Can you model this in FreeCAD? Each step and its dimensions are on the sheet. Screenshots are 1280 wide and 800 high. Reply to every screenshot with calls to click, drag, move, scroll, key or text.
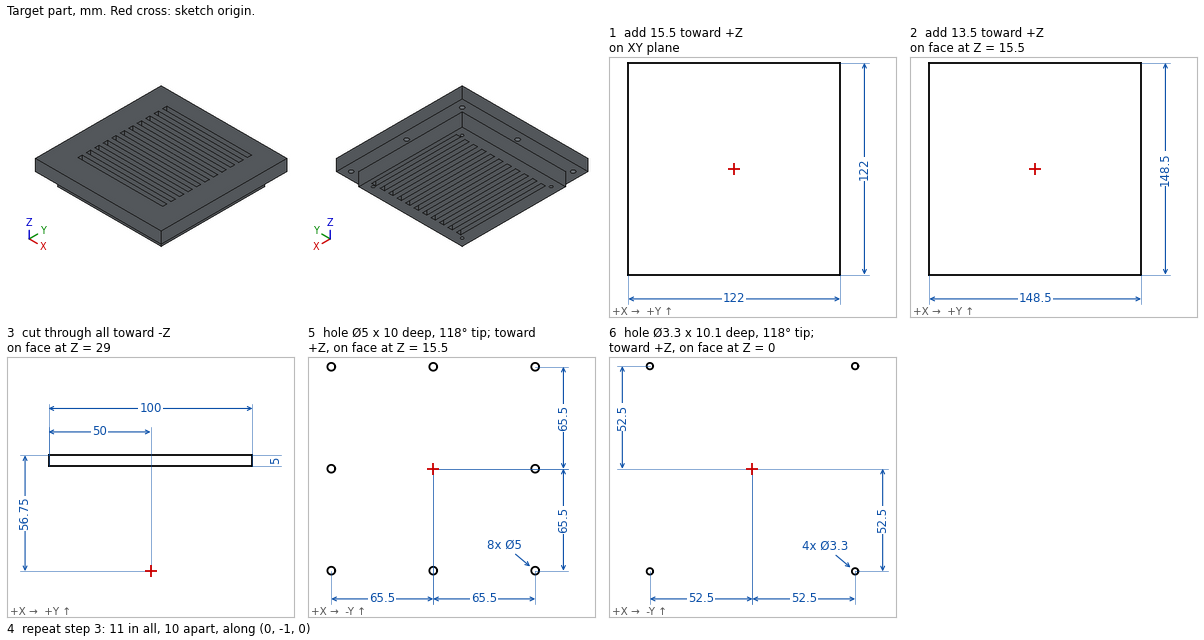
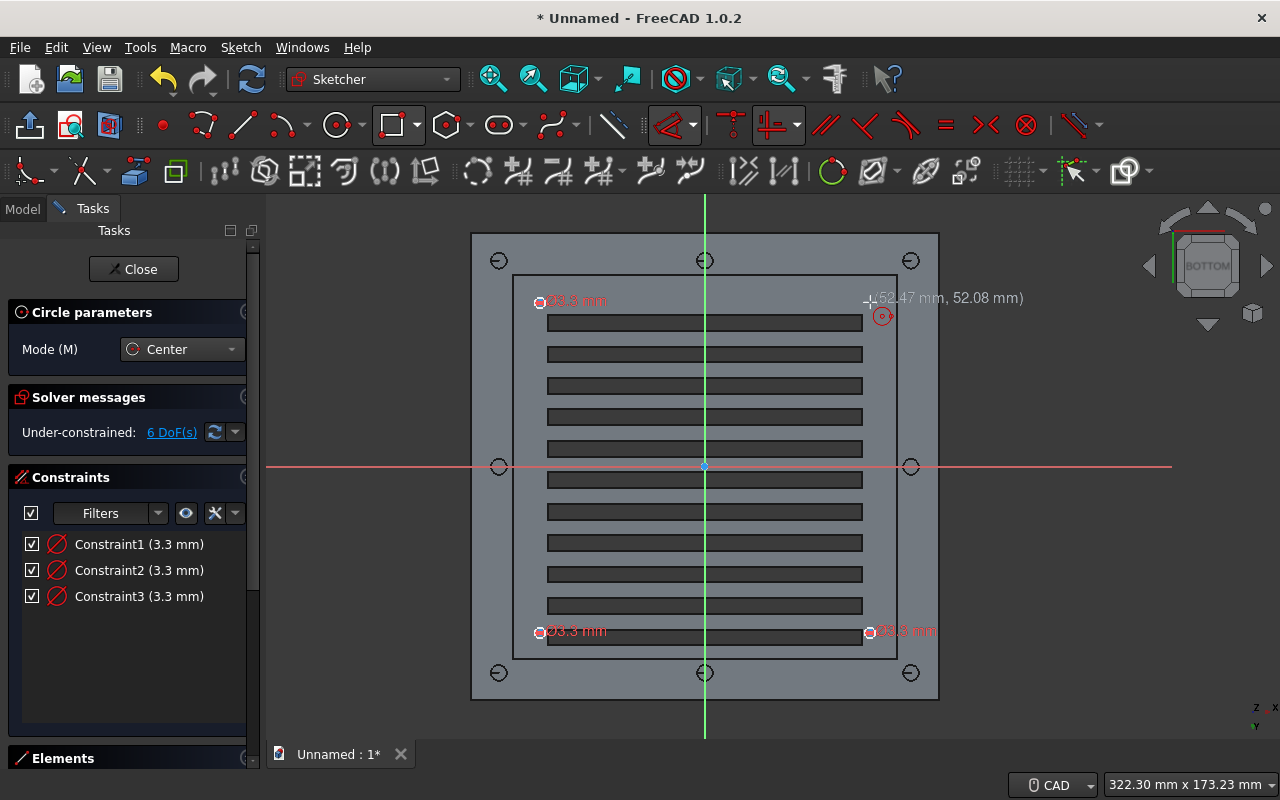
click(870, 302)
move(874, 298)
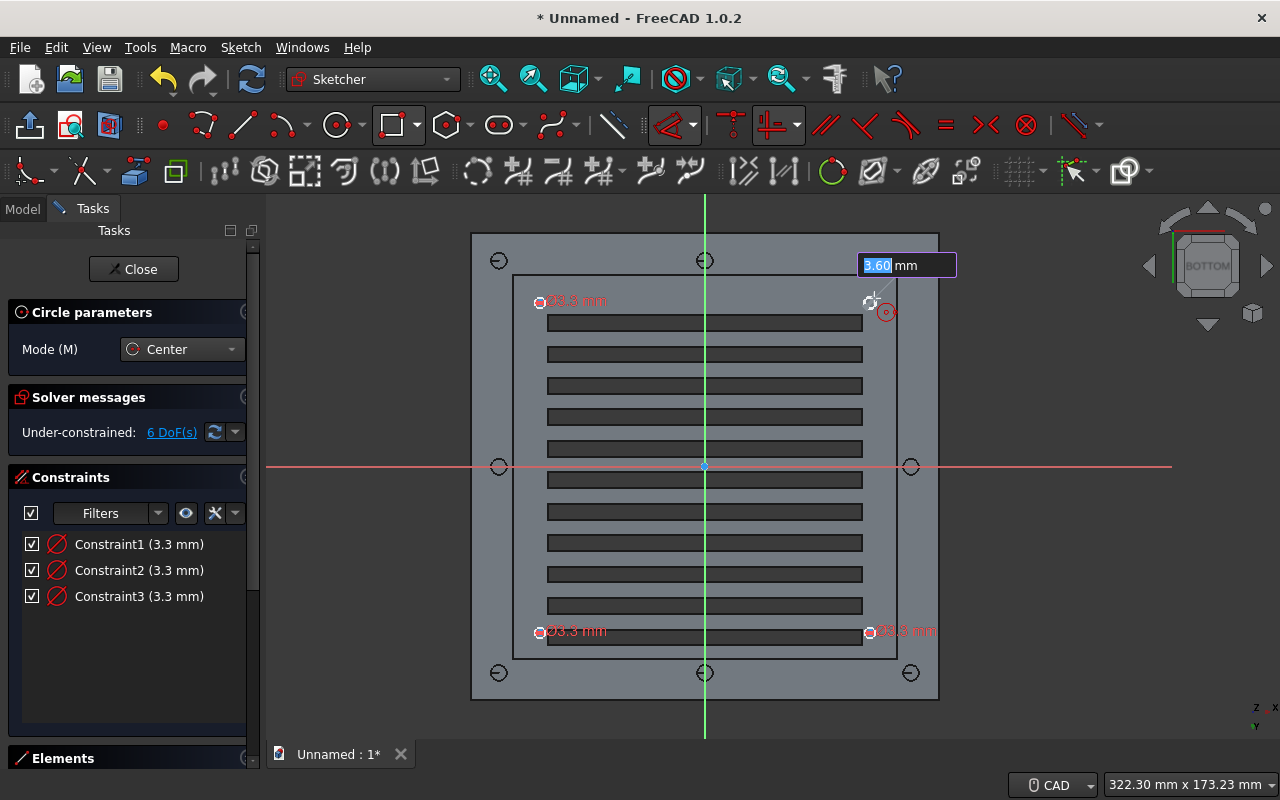
text(3.3)
key(Return)
key(Escape)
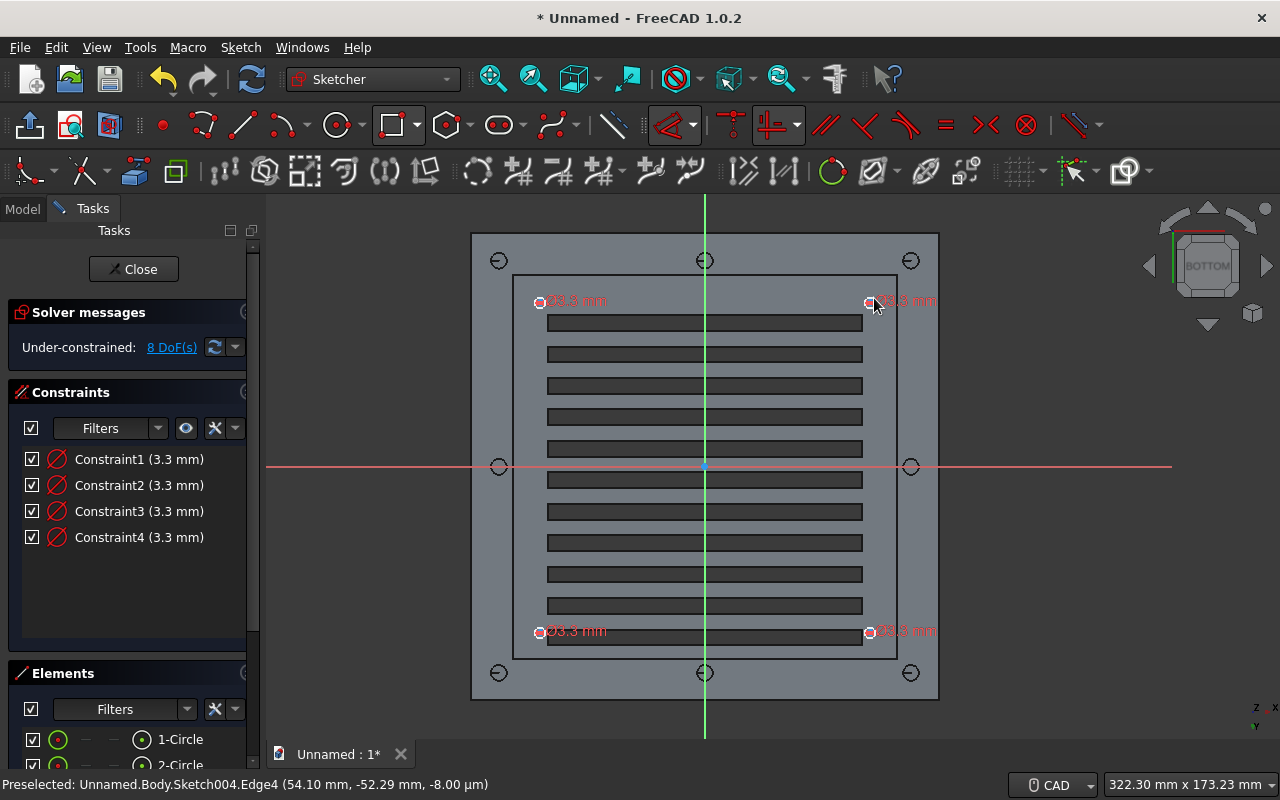
click(870, 633)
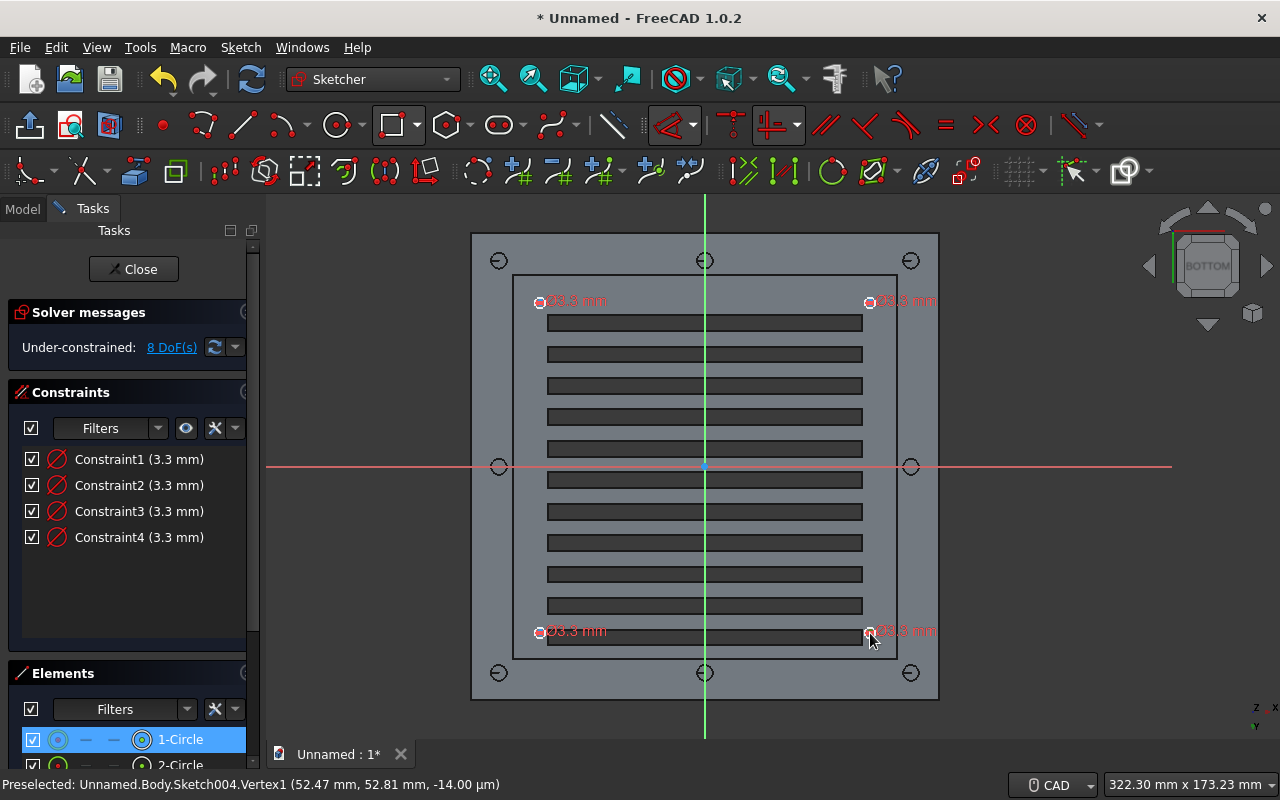
click(540, 633)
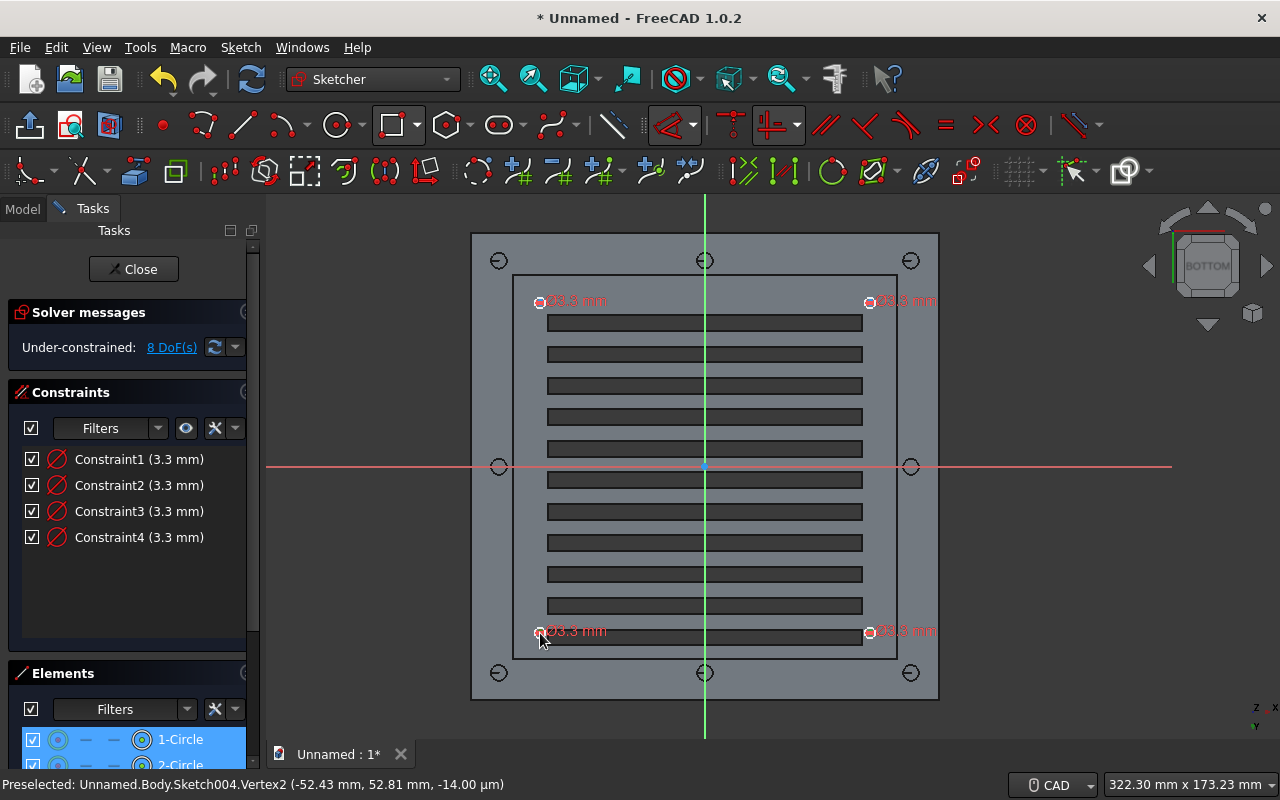
click(800, 126)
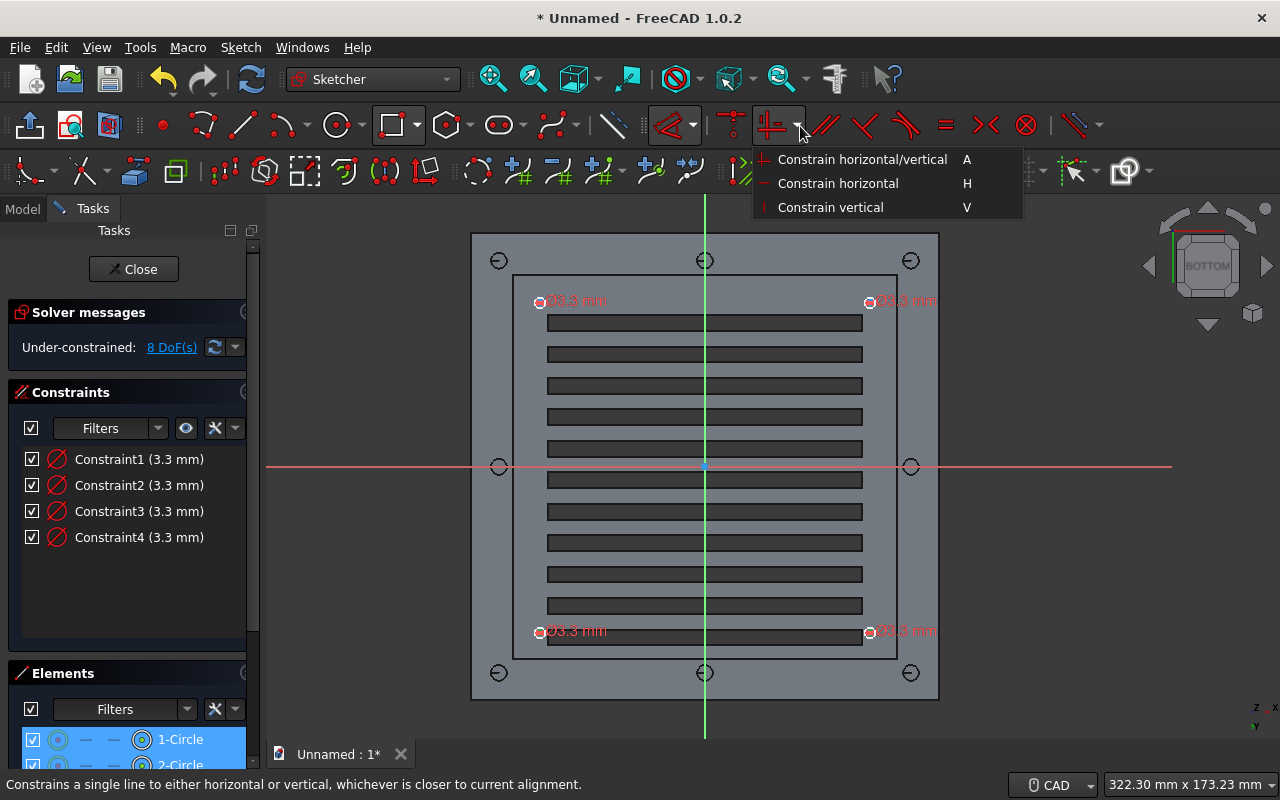
click(888, 183)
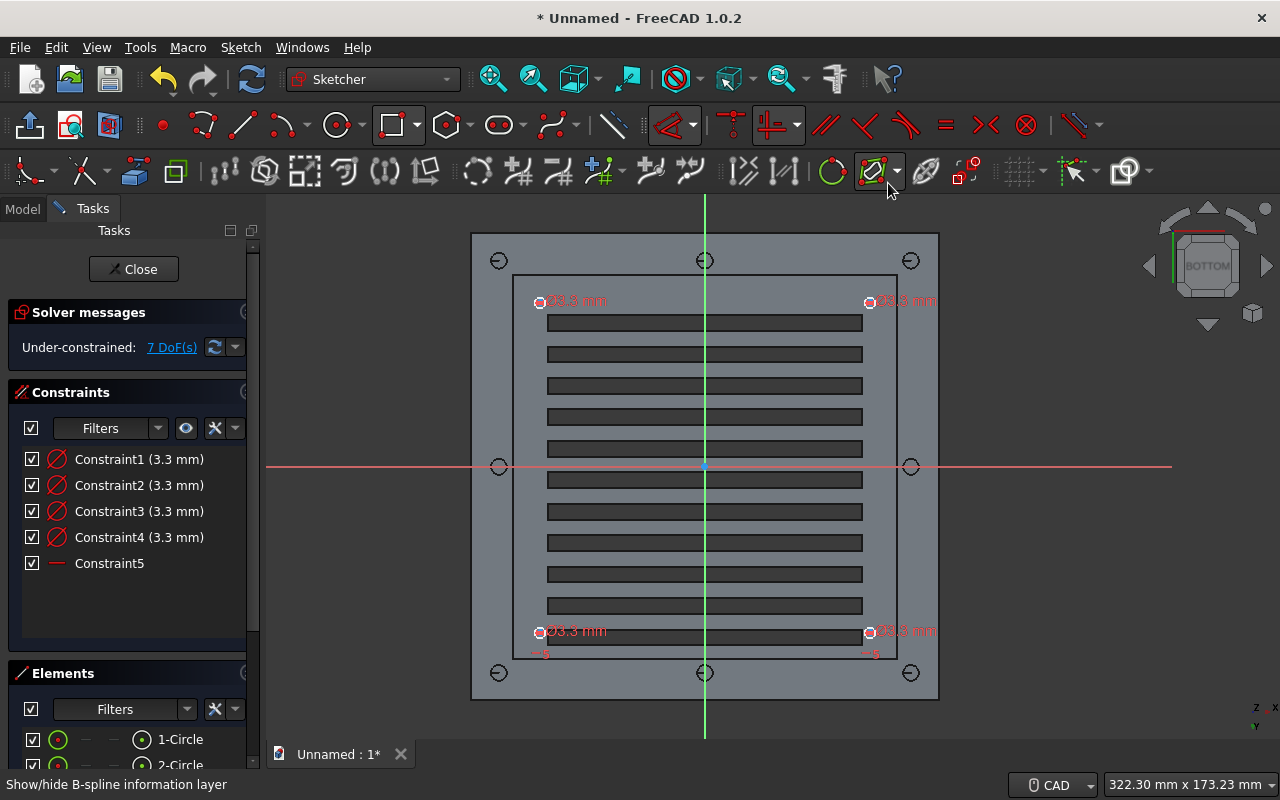
click(540, 633)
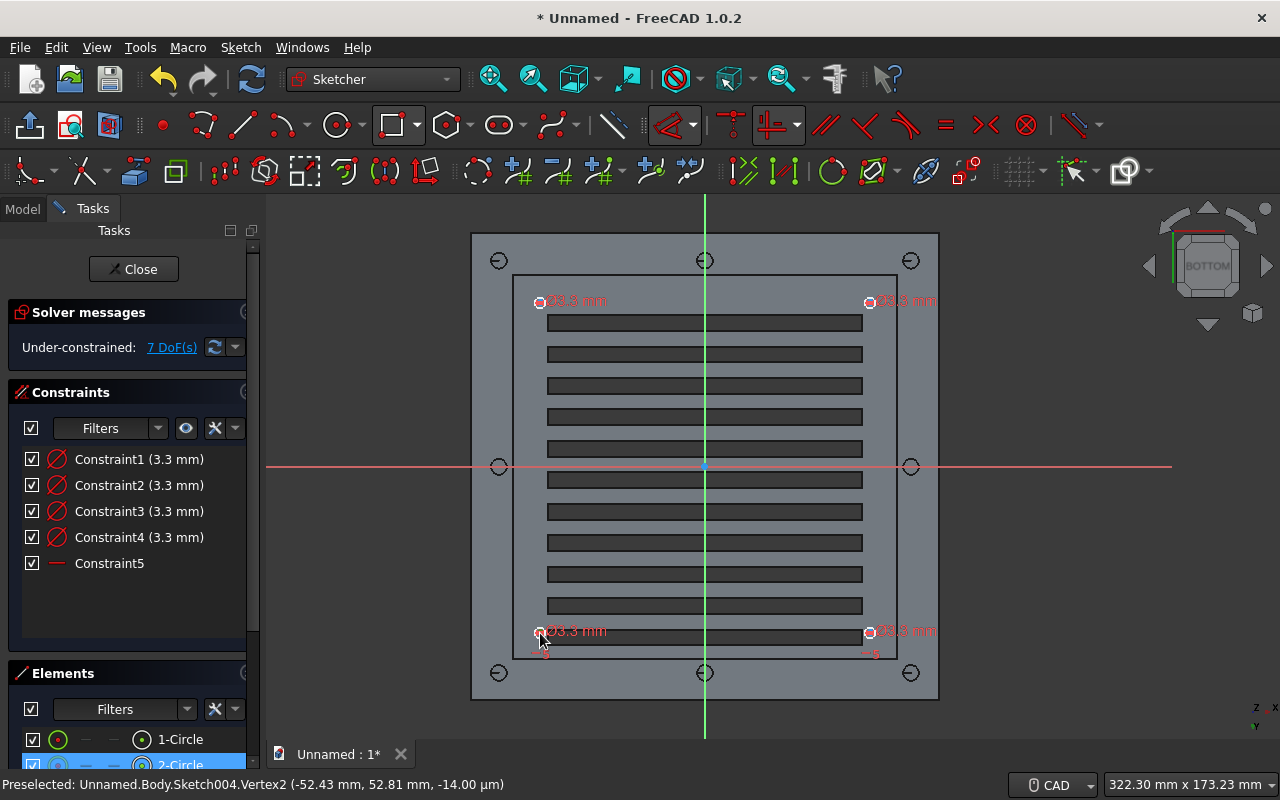
click(540, 303)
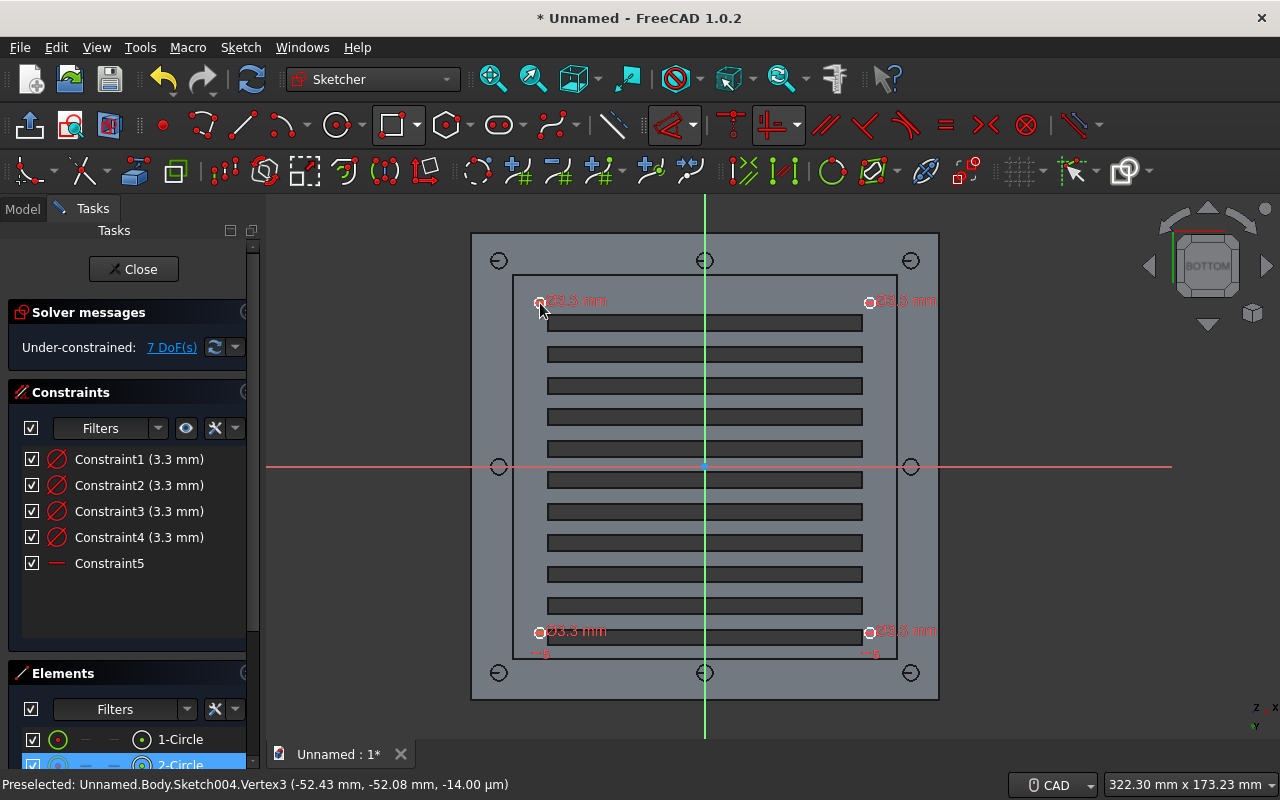
click(800, 126)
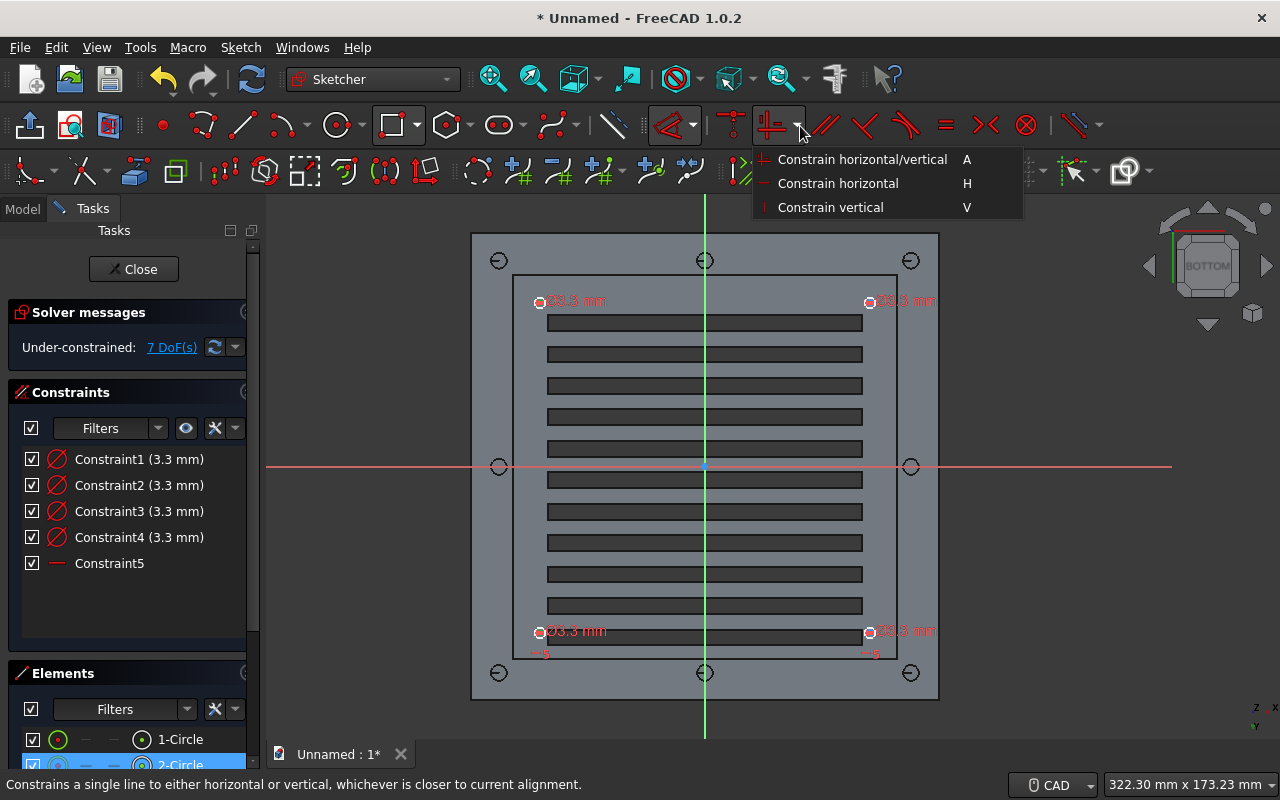
click(888, 207)